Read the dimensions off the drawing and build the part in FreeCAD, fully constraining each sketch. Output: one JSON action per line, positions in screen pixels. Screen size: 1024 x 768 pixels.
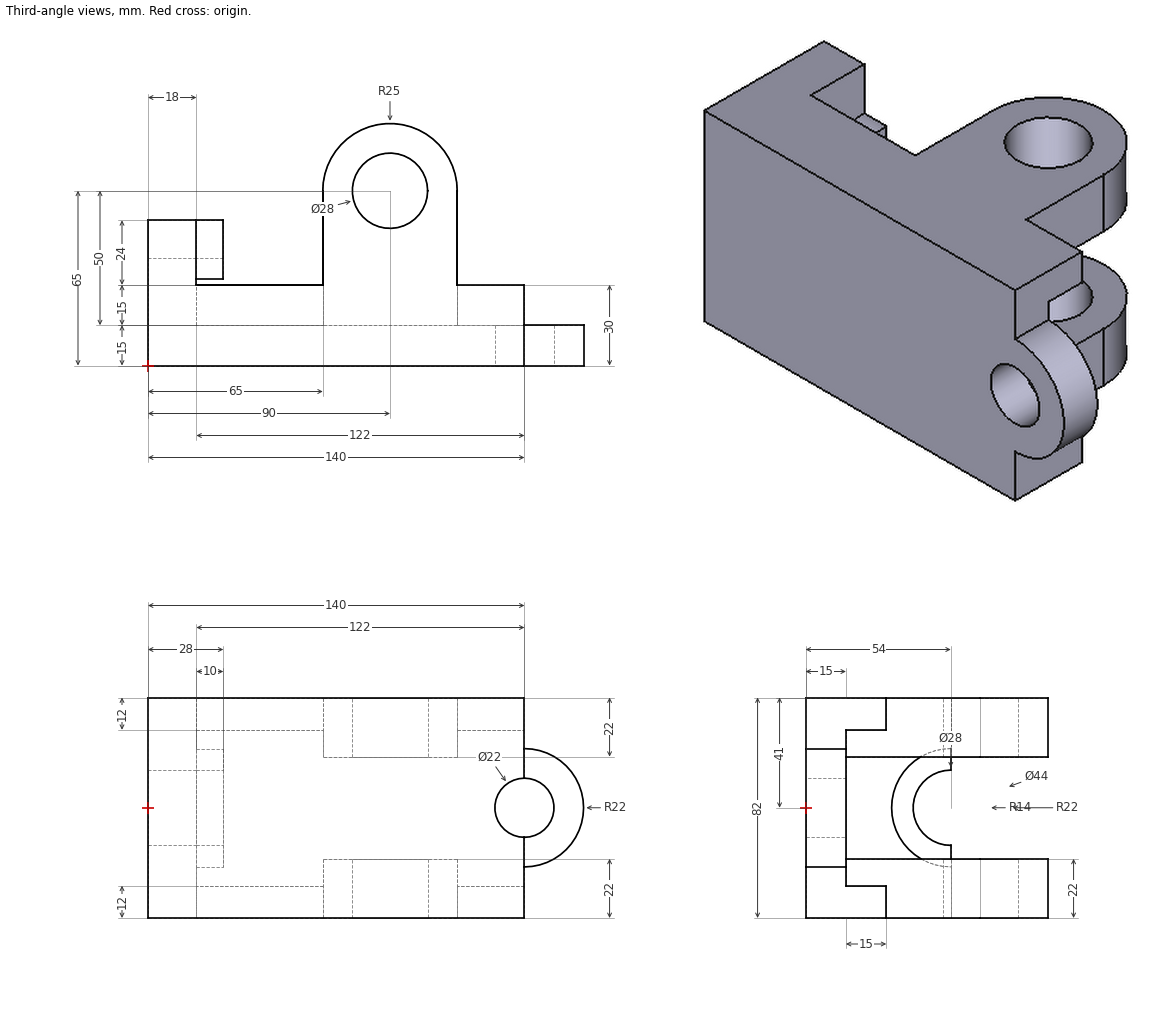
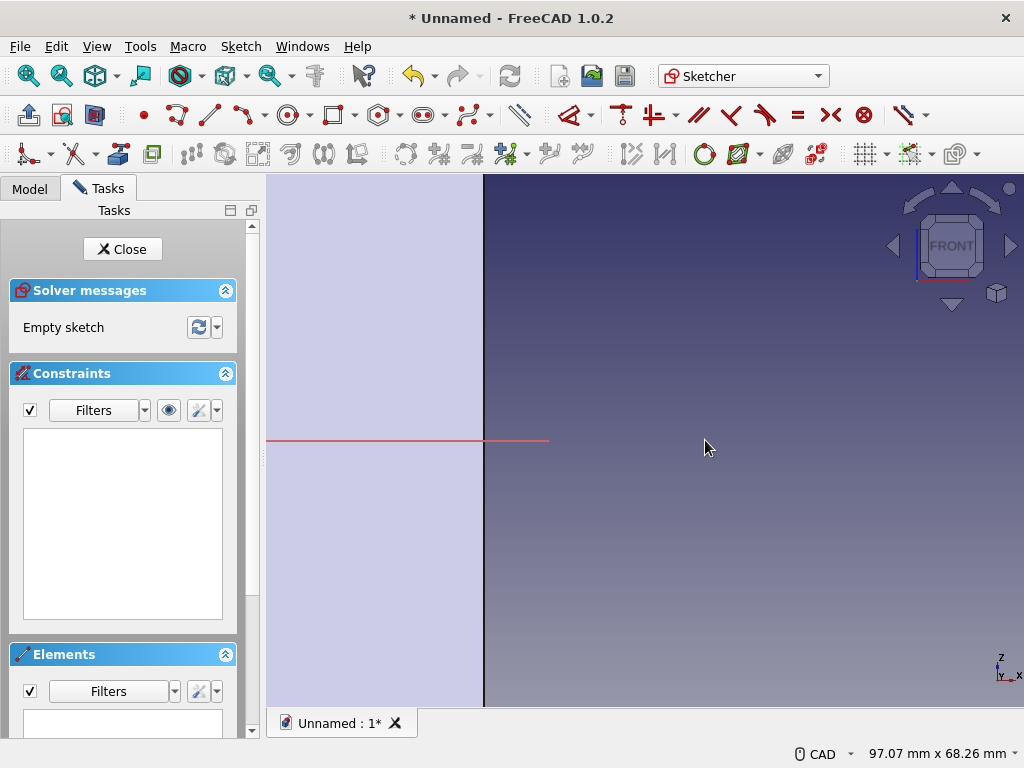
{"action": "left_click", "coordinate": [210, 116]}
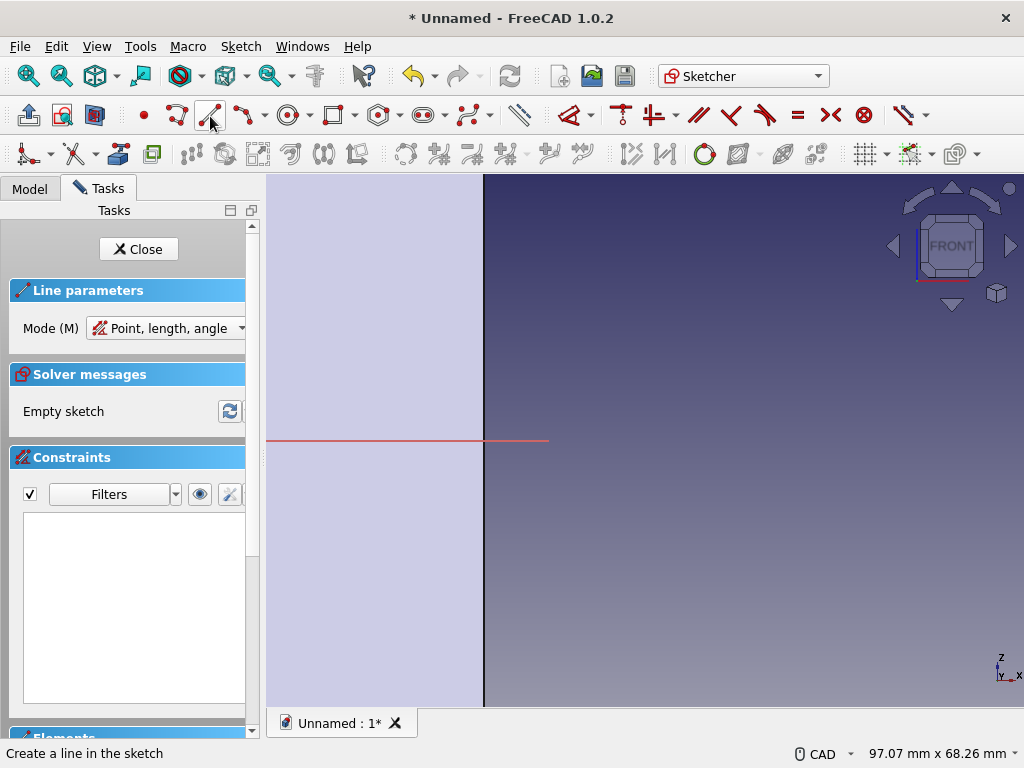
{"action": "left_click", "coordinate": [484, 269]}
{"action": "left_click", "coordinate": [484, 612]}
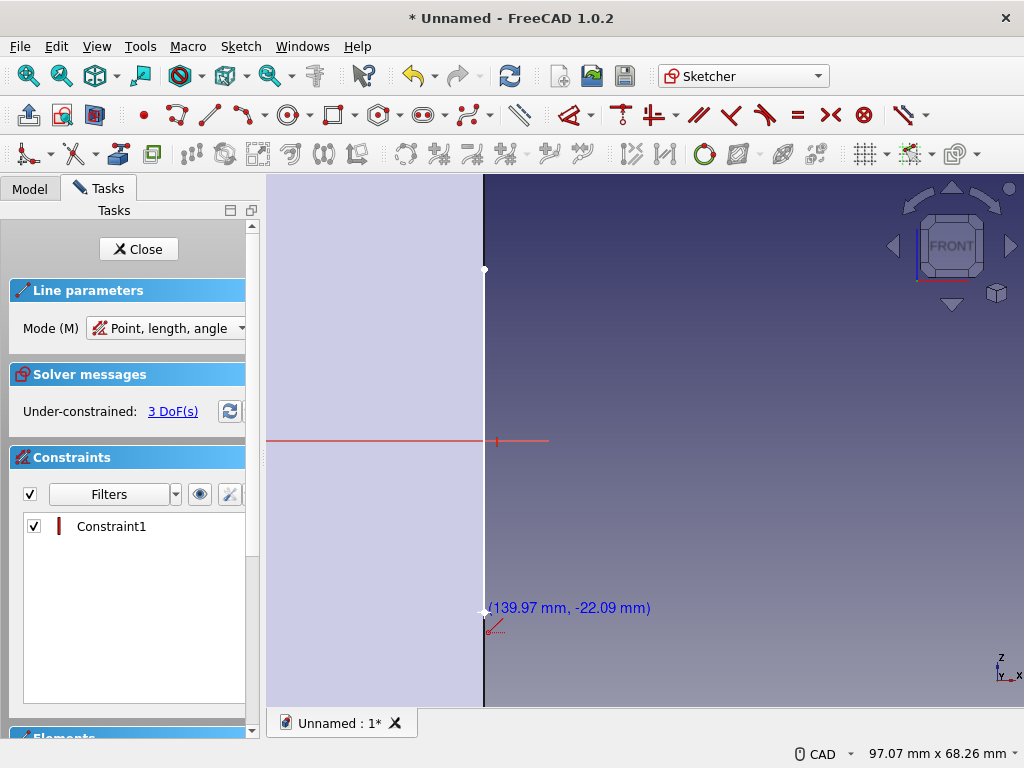
{"action": "key", "text": "g 3 a"}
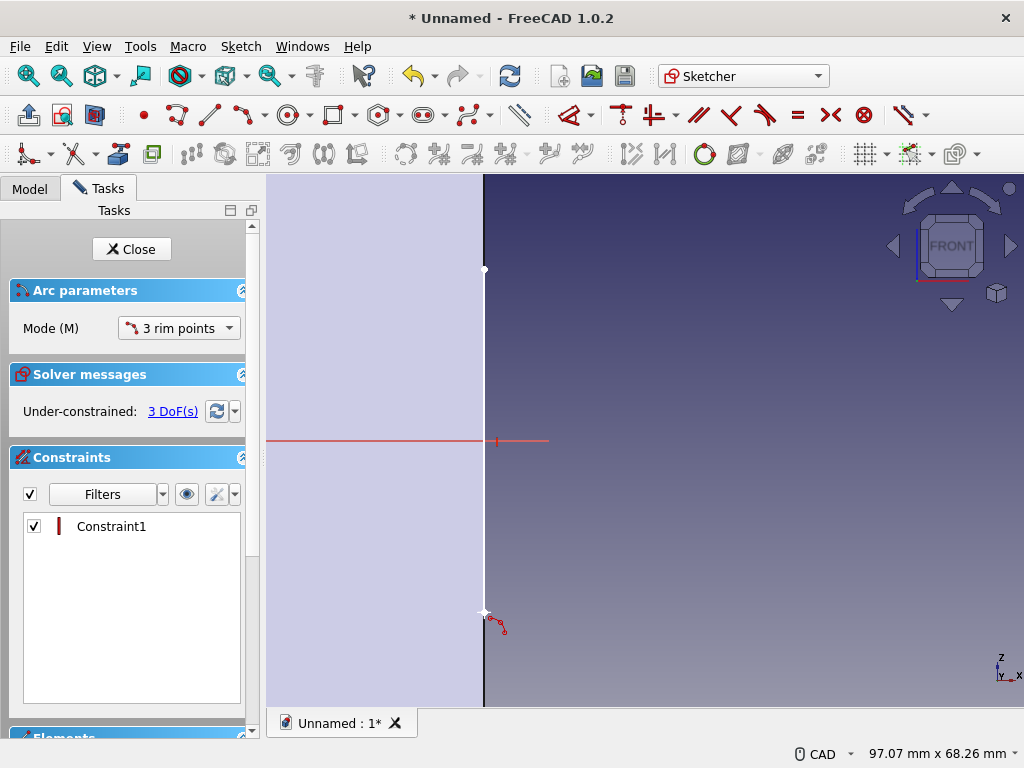
{"action": "left_click", "coordinate": [484, 613]}
{"action": "left_click", "coordinate": [484, 270]}
{"action": "left_click", "coordinate": [648, 494]}
{"action": "key", "text": "Escape"}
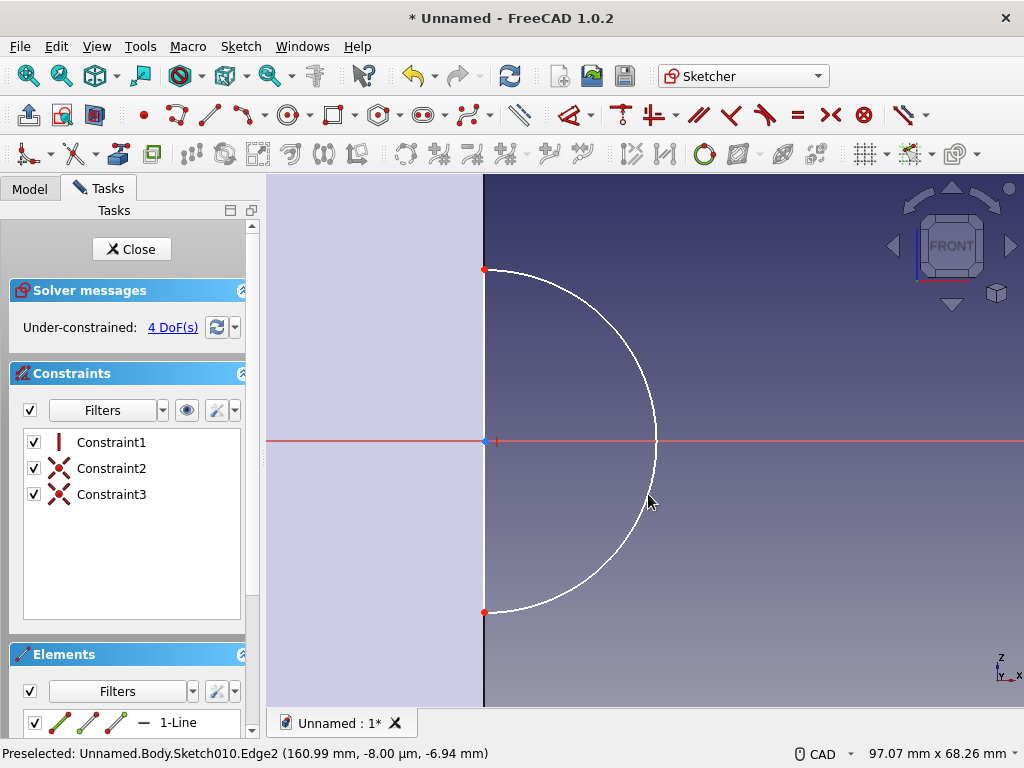
{"action": "left_click", "coordinate": [485, 442]}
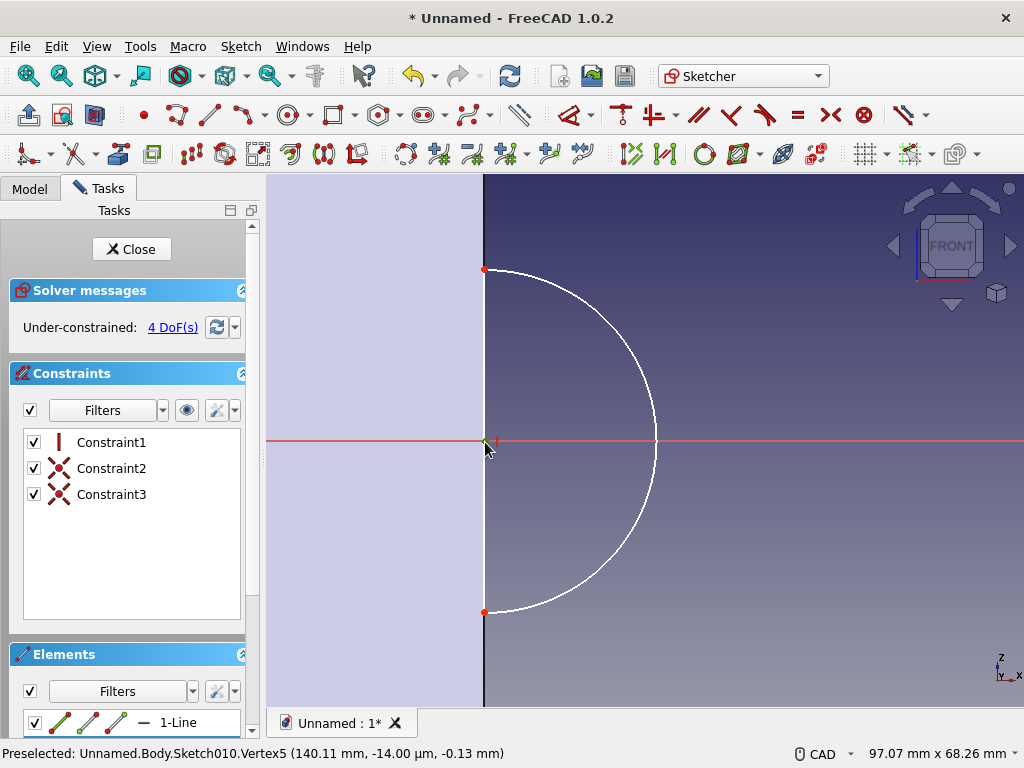
{"action": "left_click", "coordinate": [334, 440]}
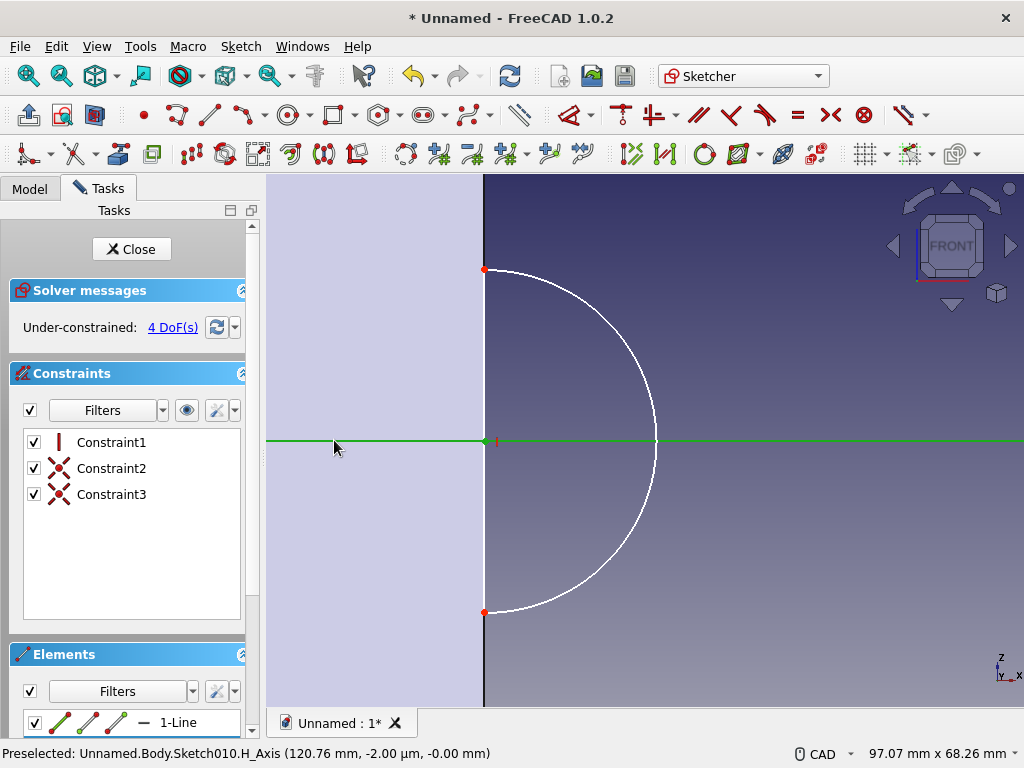
{"action": "key", "text": "c"}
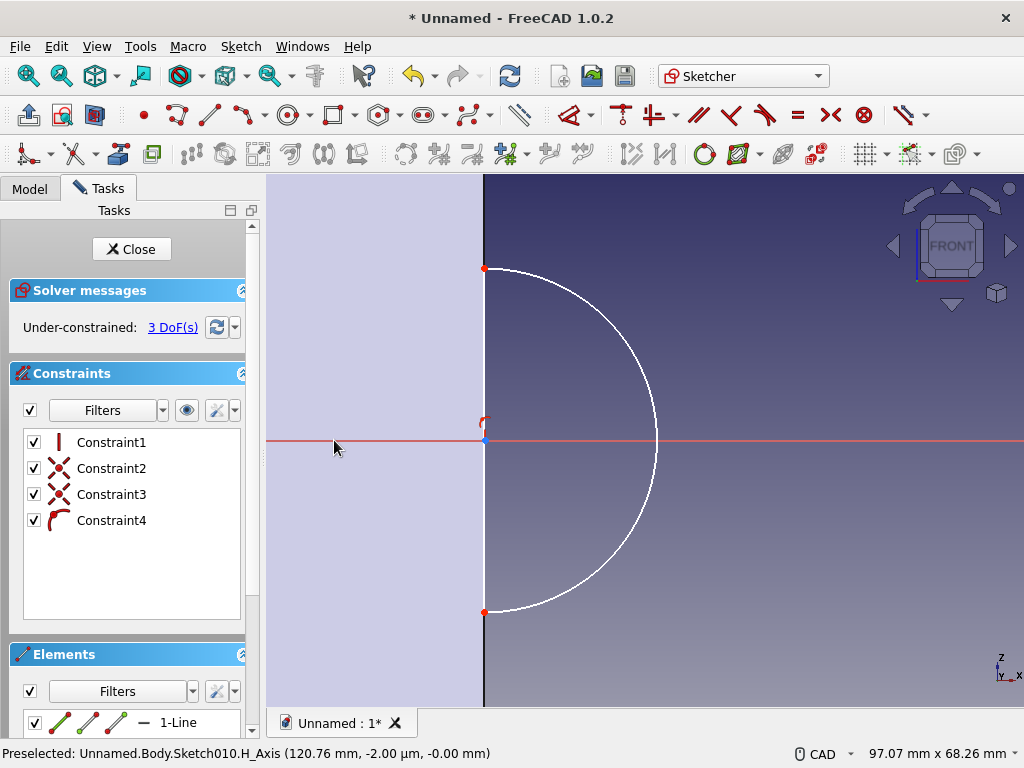
{"action": "key", "text": "d"}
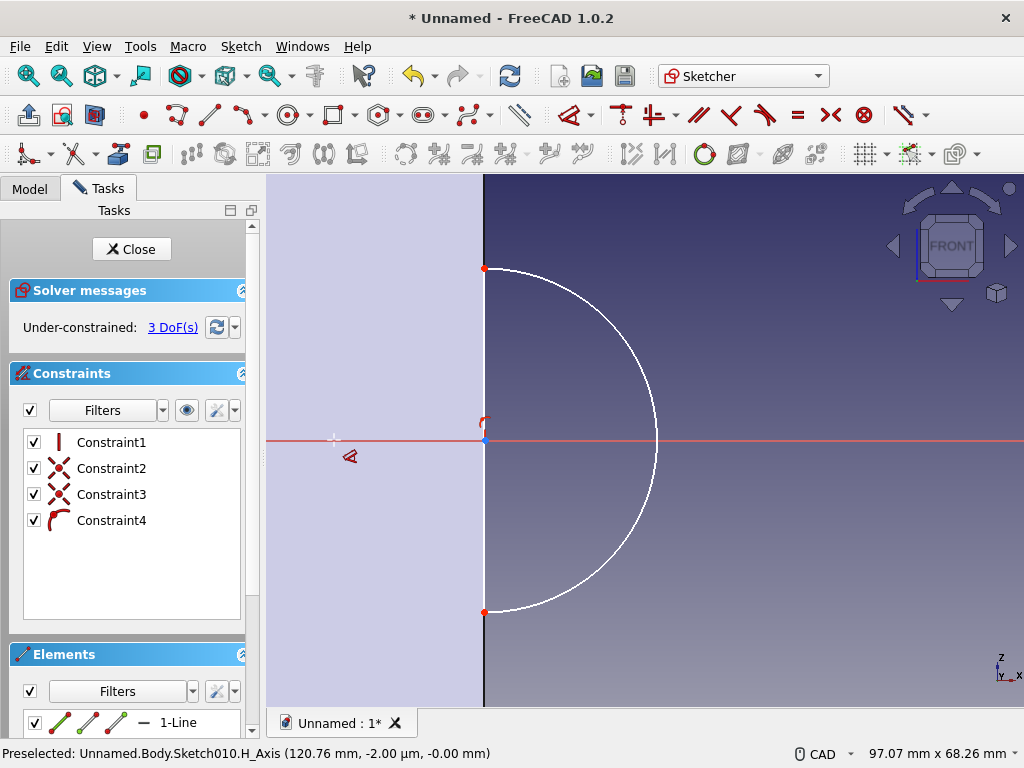
{"action": "left_click", "coordinate": [624, 542]}
{"action": "left_click", "coordinate": [650, 561]}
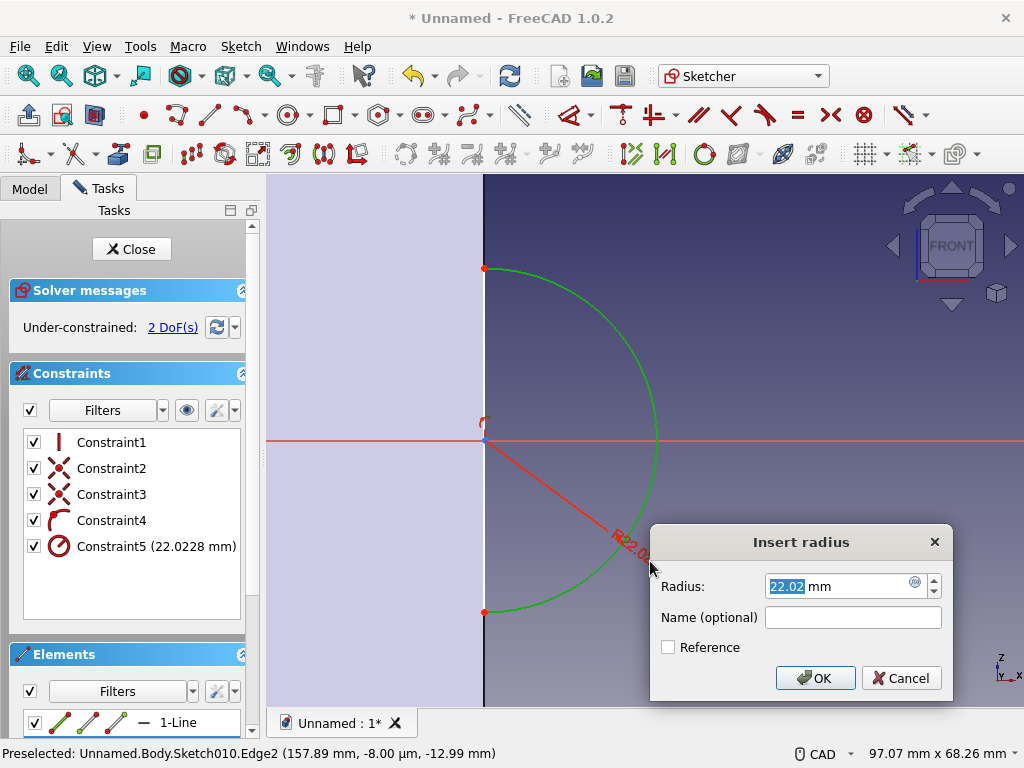
{"action": "type", "text": "22"}
{"action": "key", "text": "Return"}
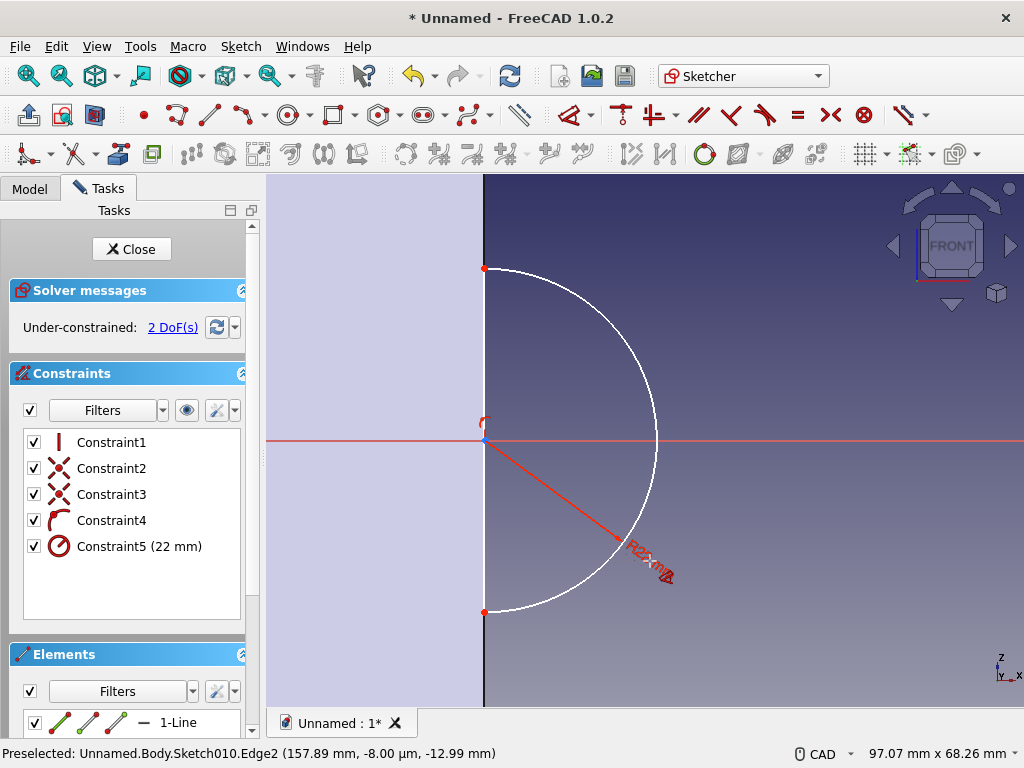
{"action": "left_click", "coordinate": [484, 269]}
{"action": "left_click", "coordinate": [389, 235]}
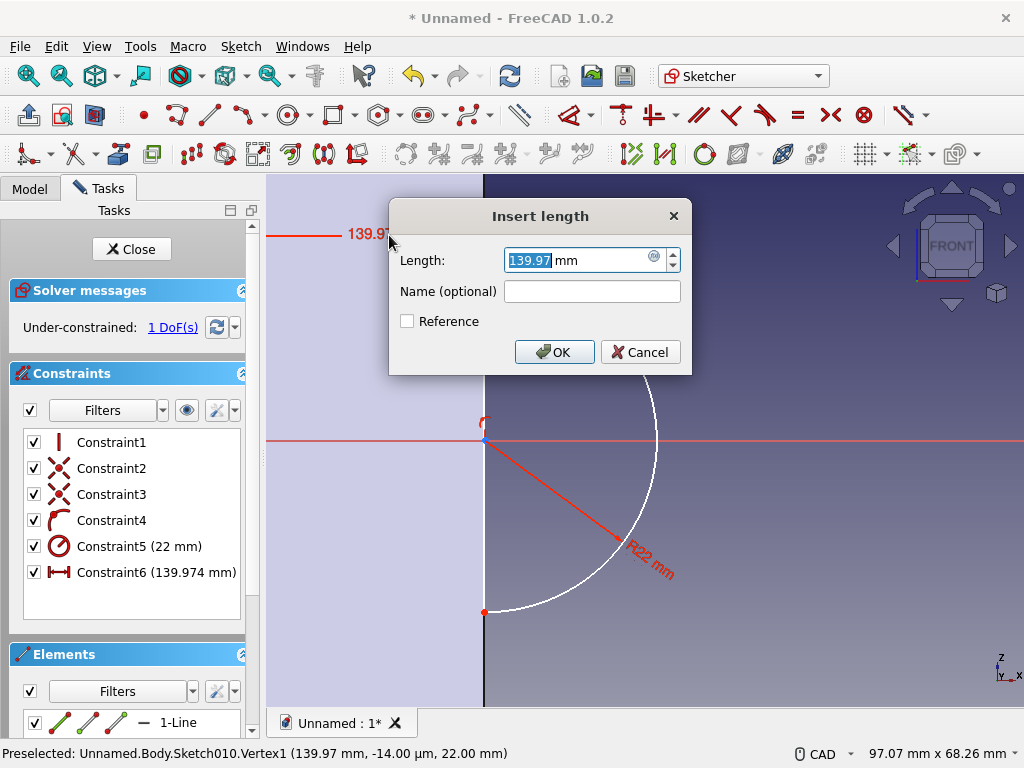
{"action": "type", "text": "140"}
{"action": "key", "text": "Return"}